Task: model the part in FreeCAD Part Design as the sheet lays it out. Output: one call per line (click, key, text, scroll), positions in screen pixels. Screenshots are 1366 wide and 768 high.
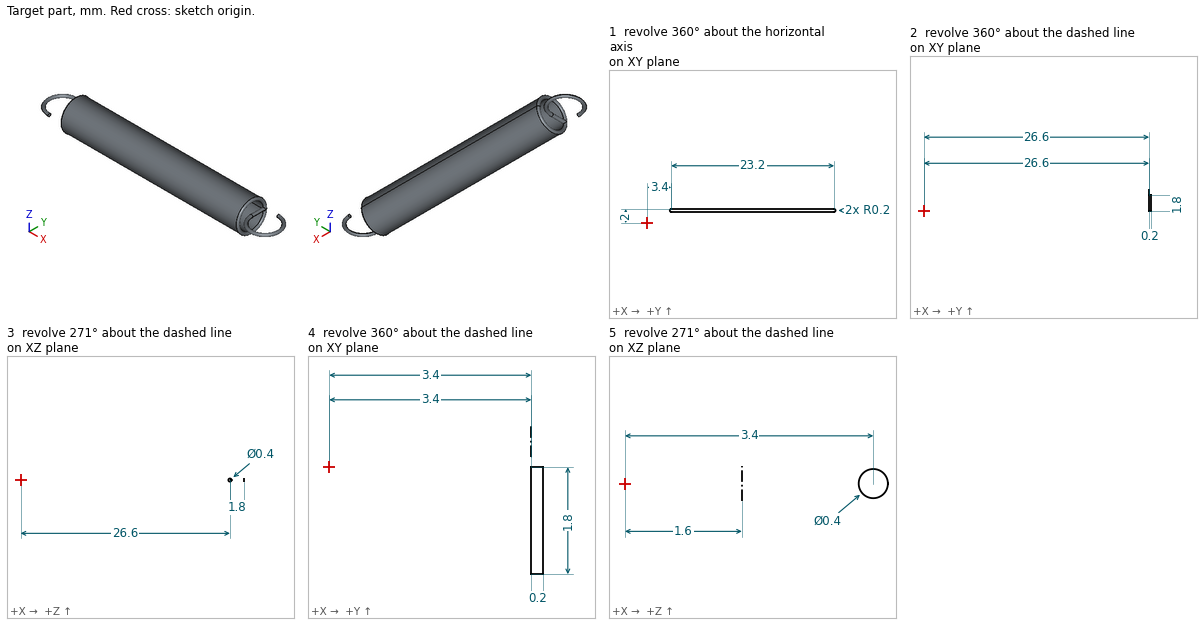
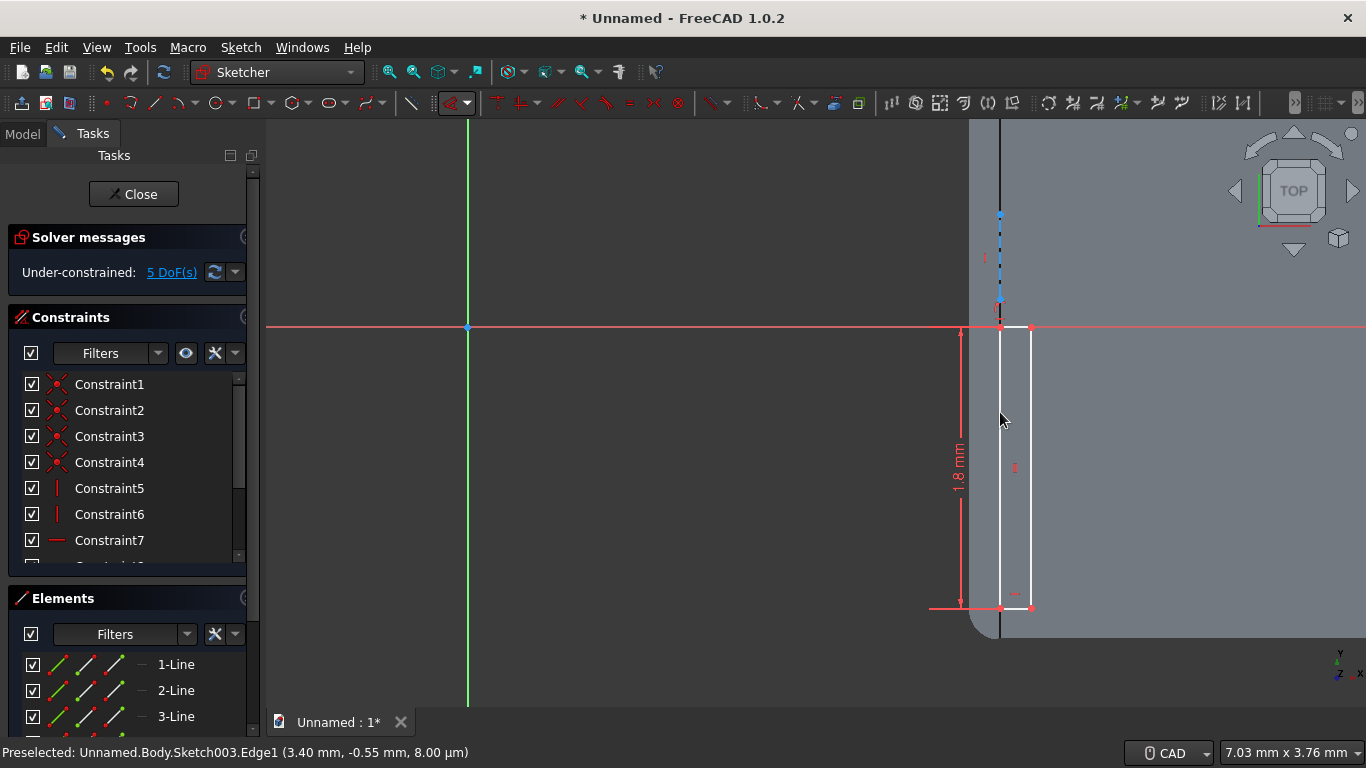
scroll(1009, 609, up, 2)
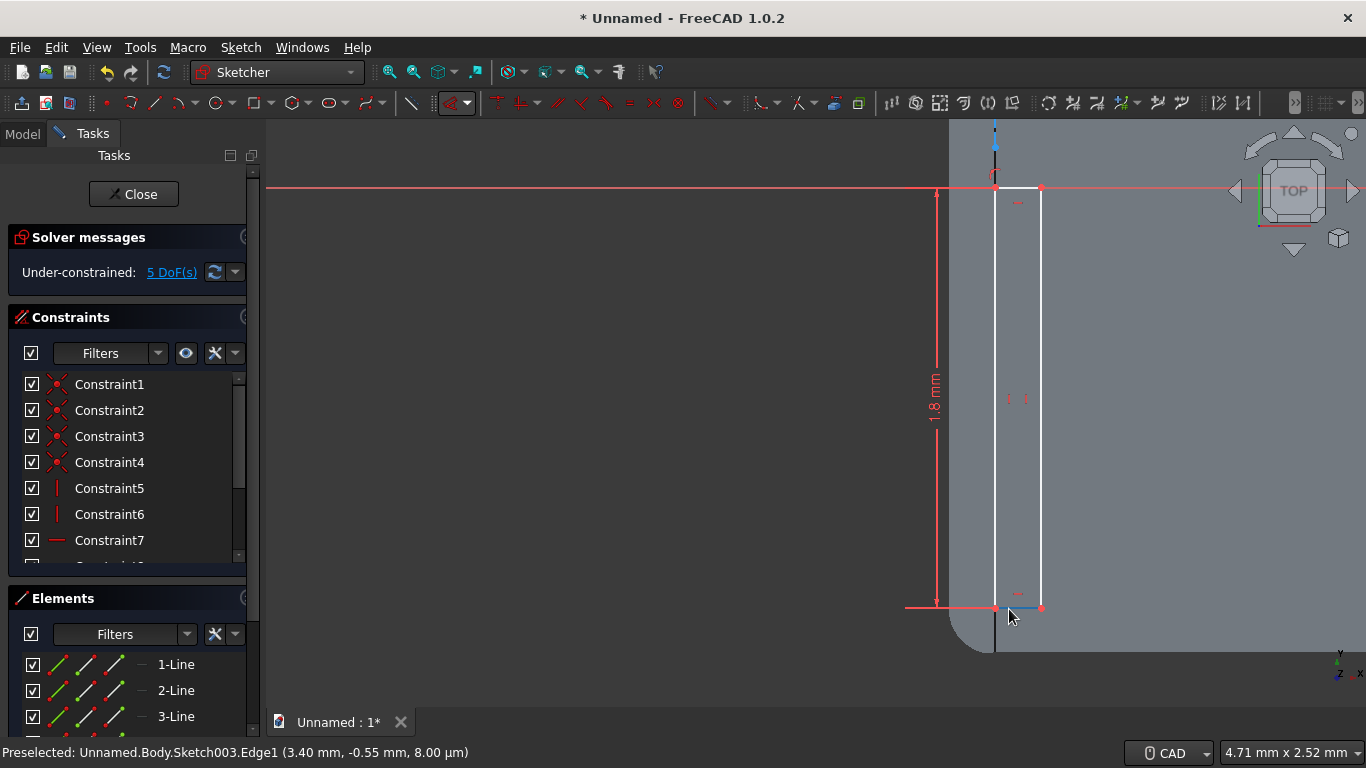
click(1009, 608)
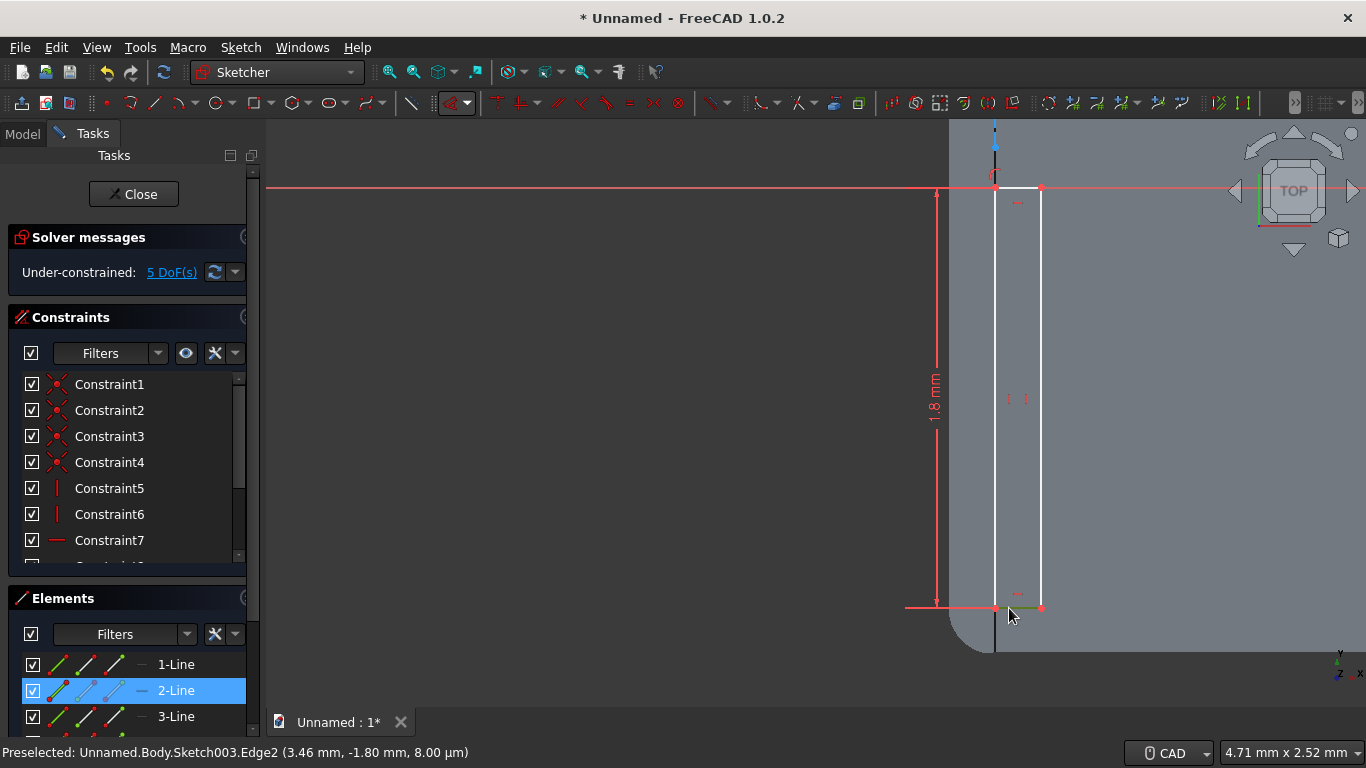
key(l)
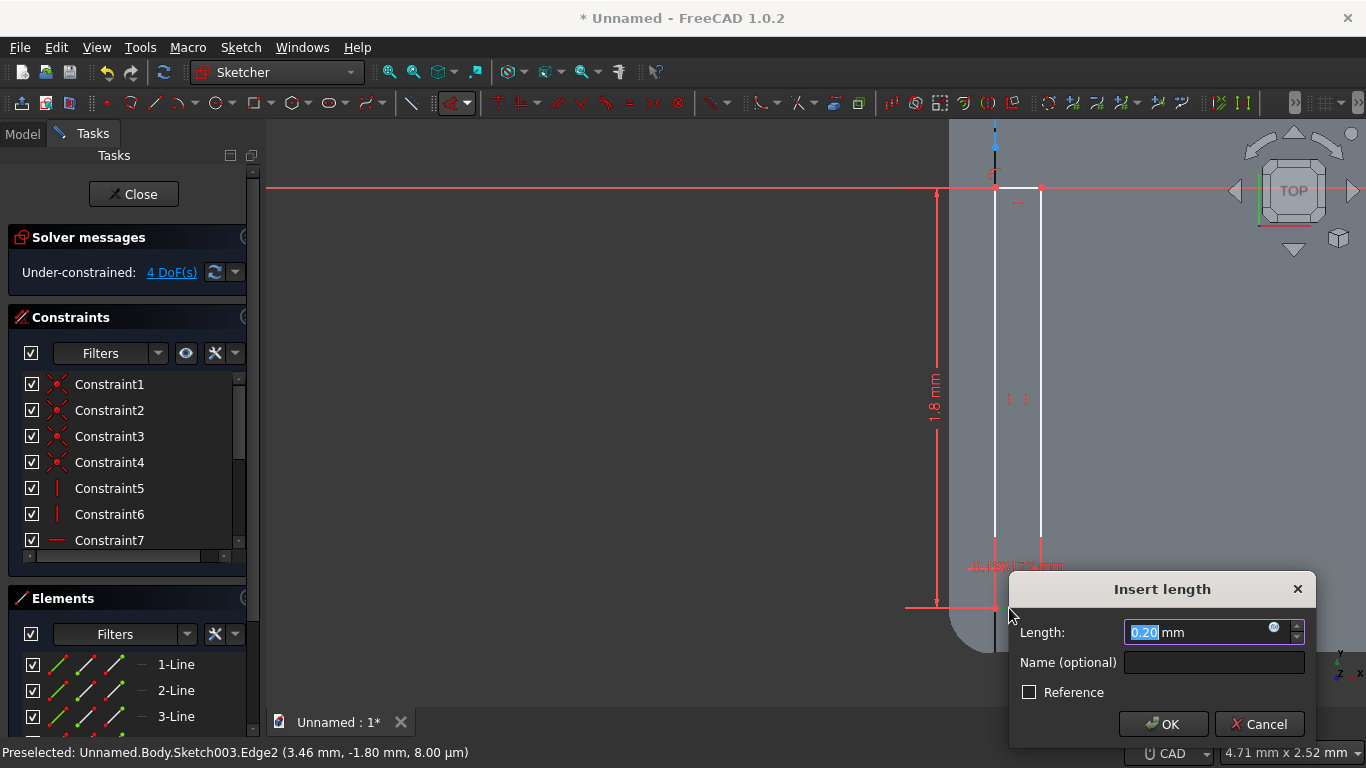
text(0.2)
key(Return)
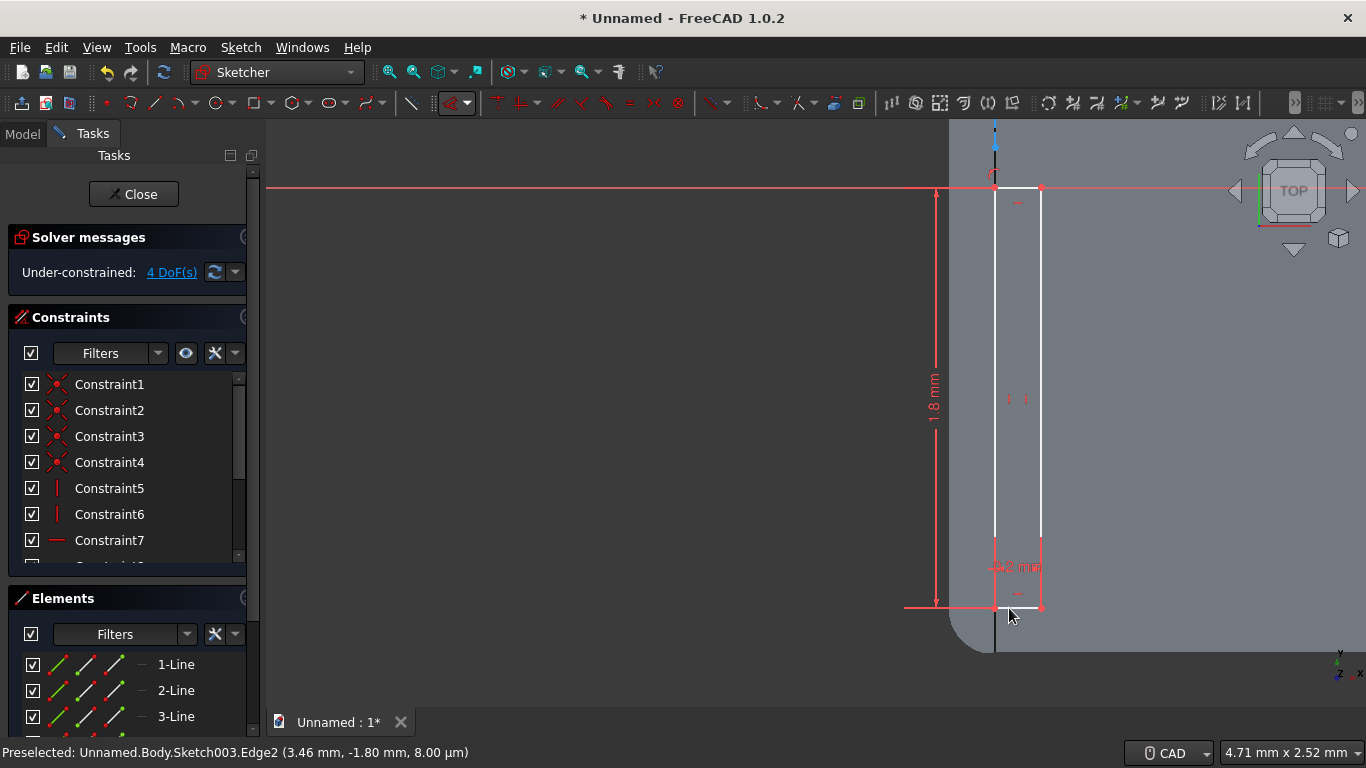
click(995, 188)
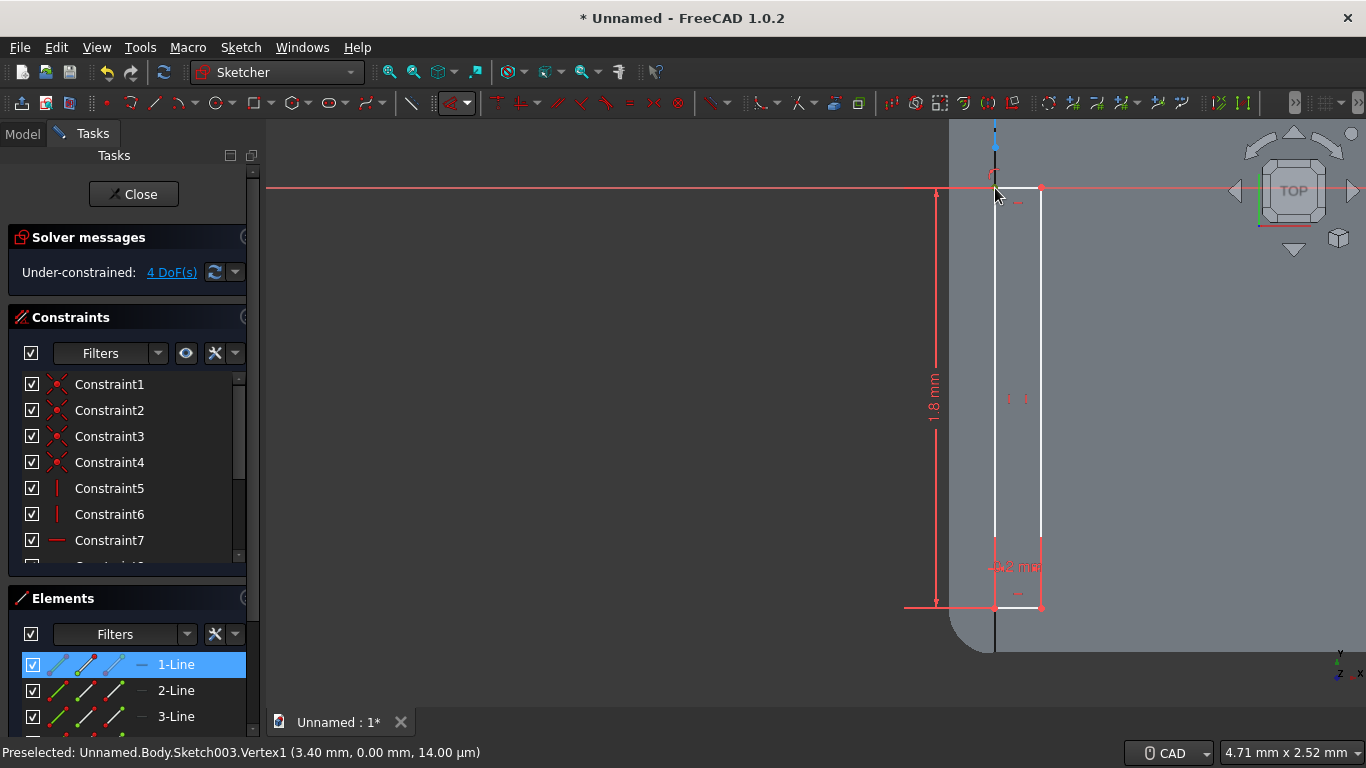
key(l)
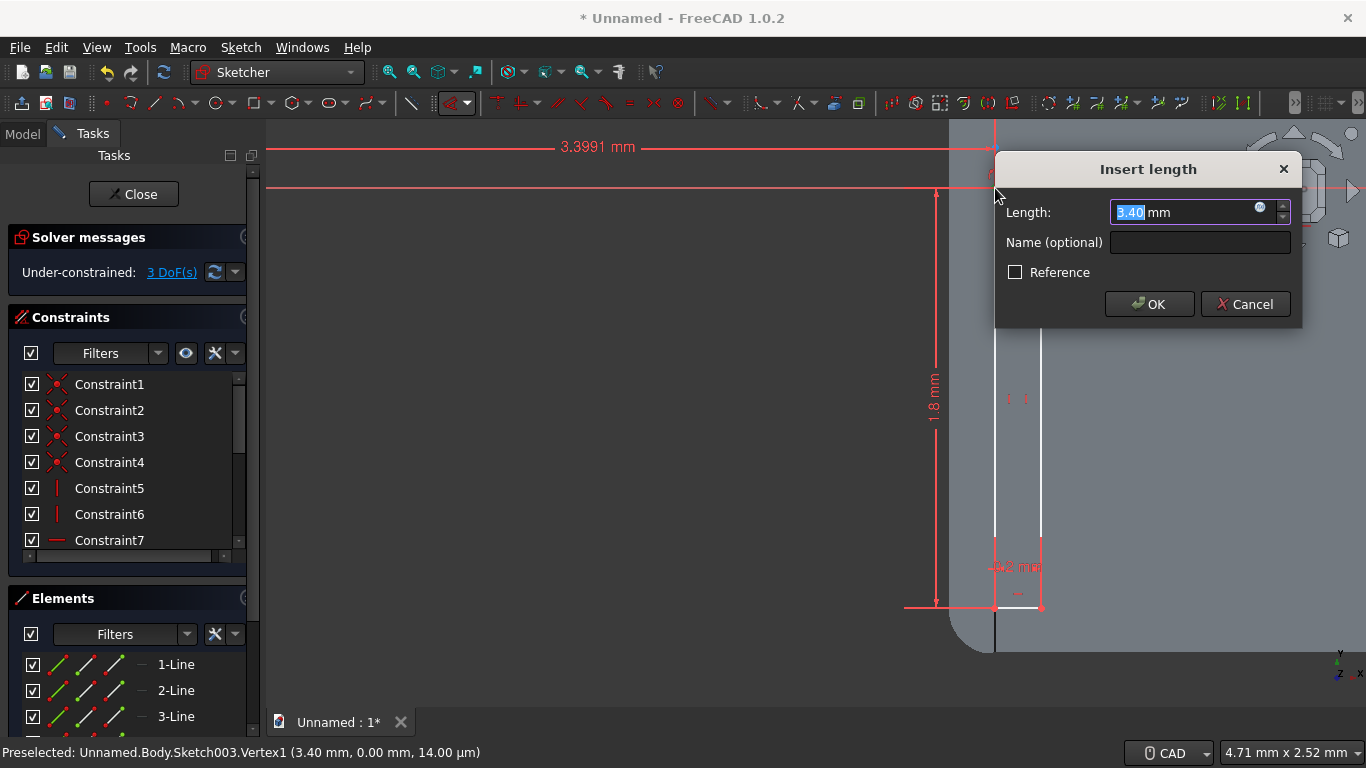
text(3.4)
key(Return)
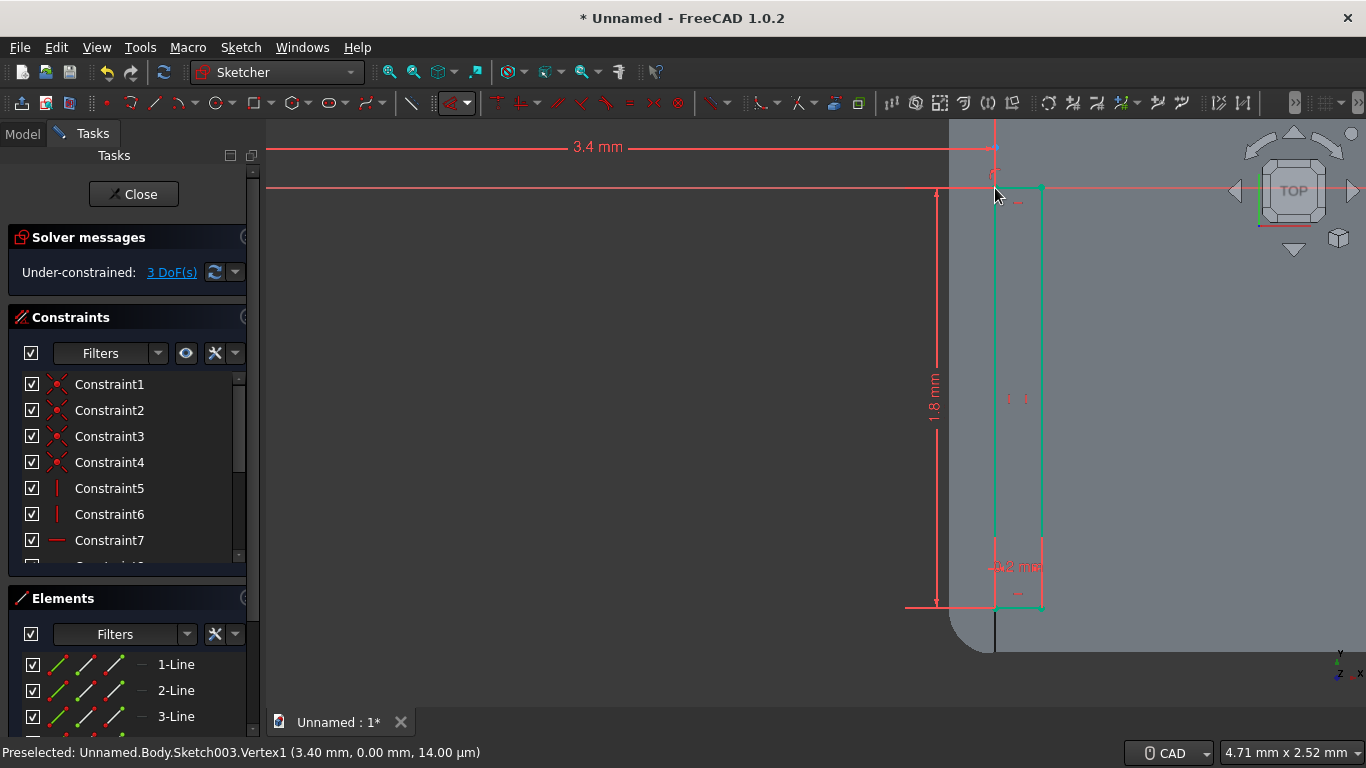
click(995, 148)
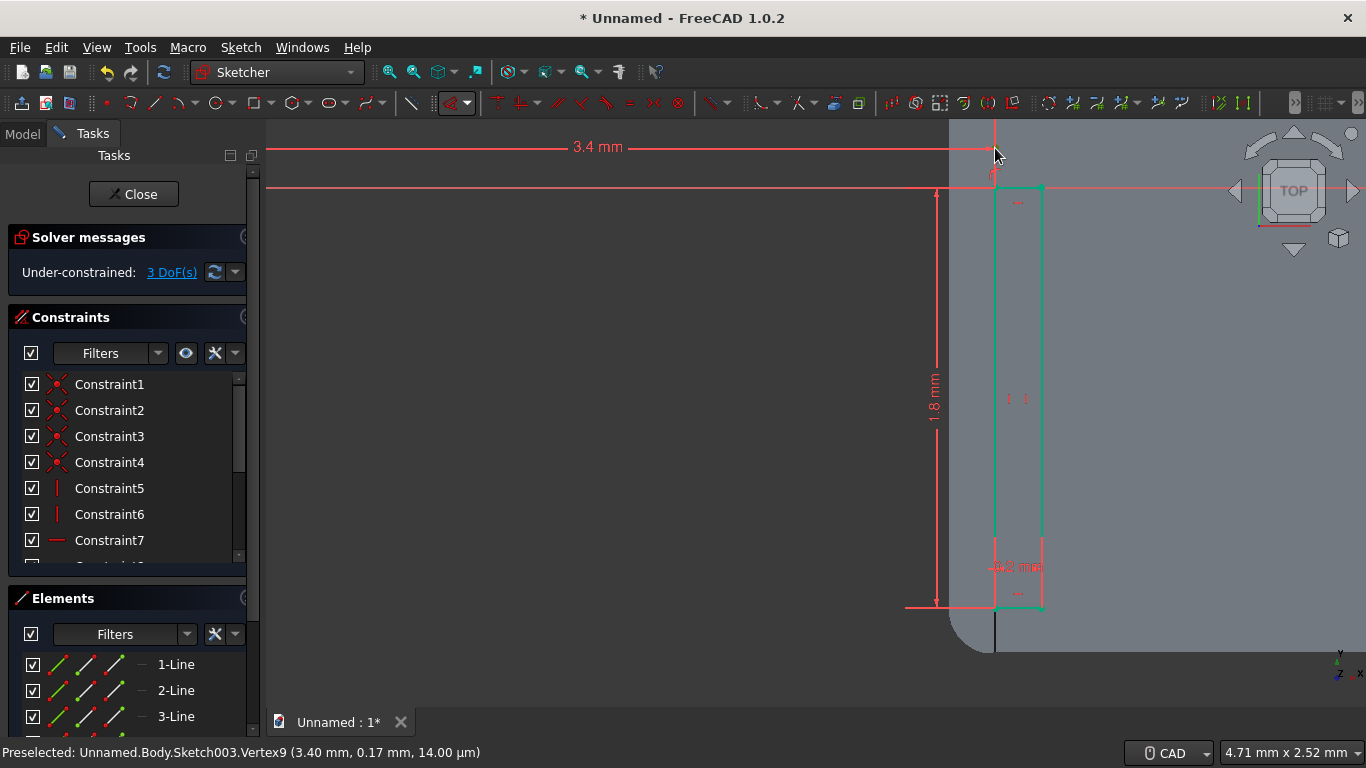
click(470, 104)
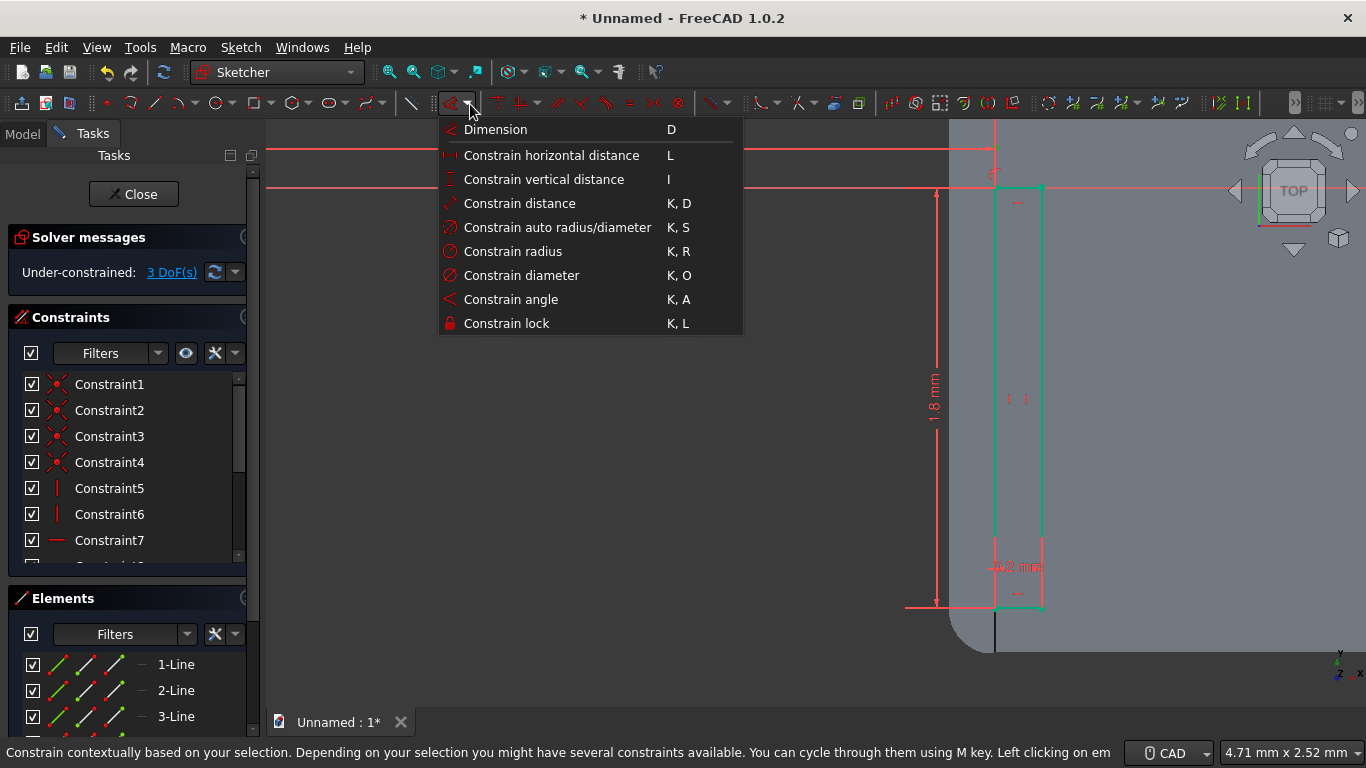
click(591, 155)